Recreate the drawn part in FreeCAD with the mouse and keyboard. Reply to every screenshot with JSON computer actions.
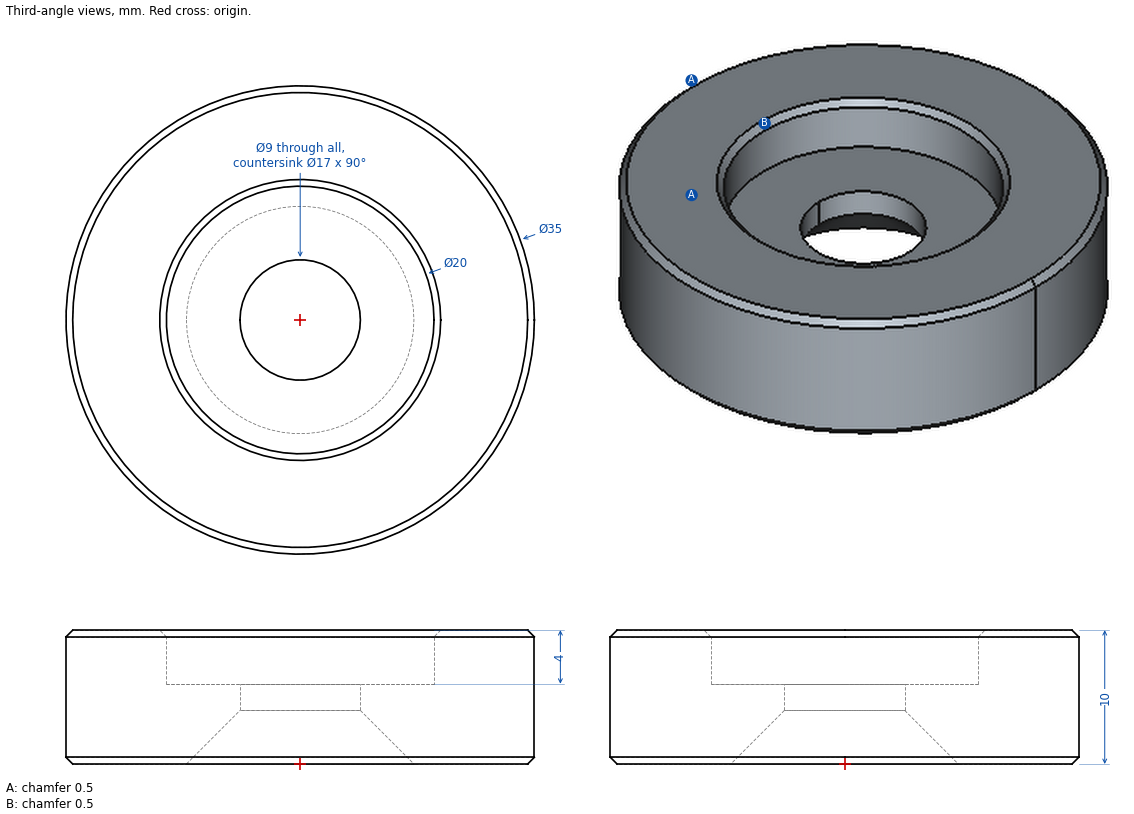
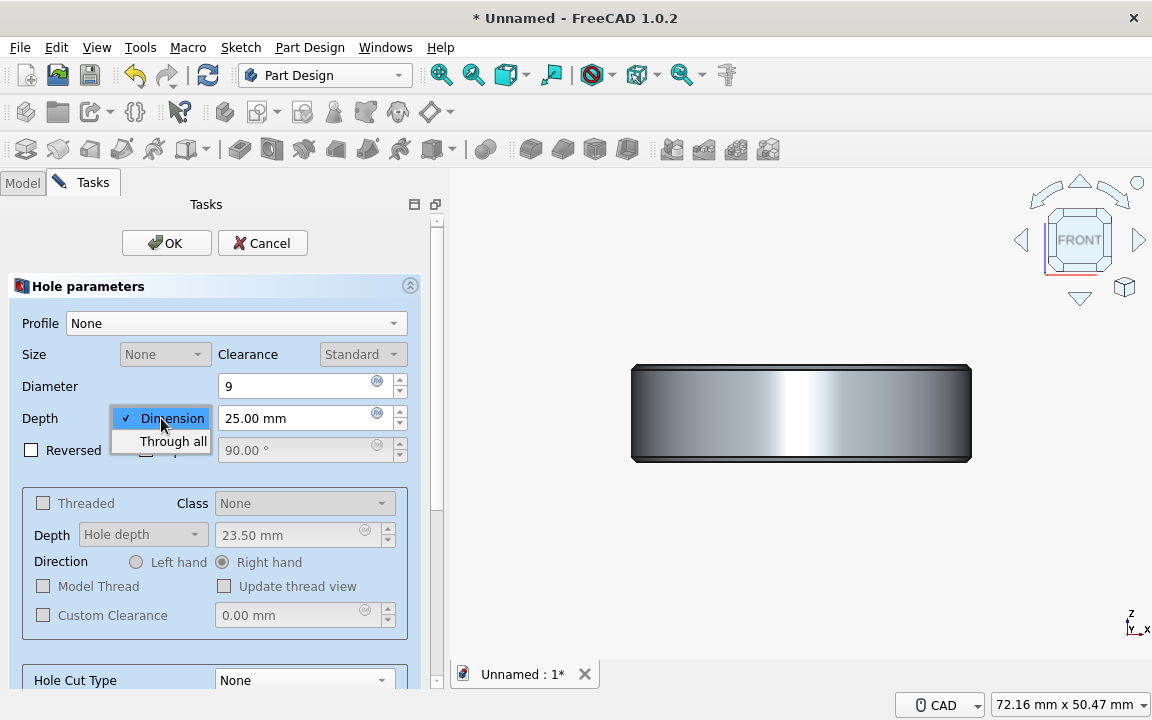
{"action": "left_click", "coordinate": [160, 442]}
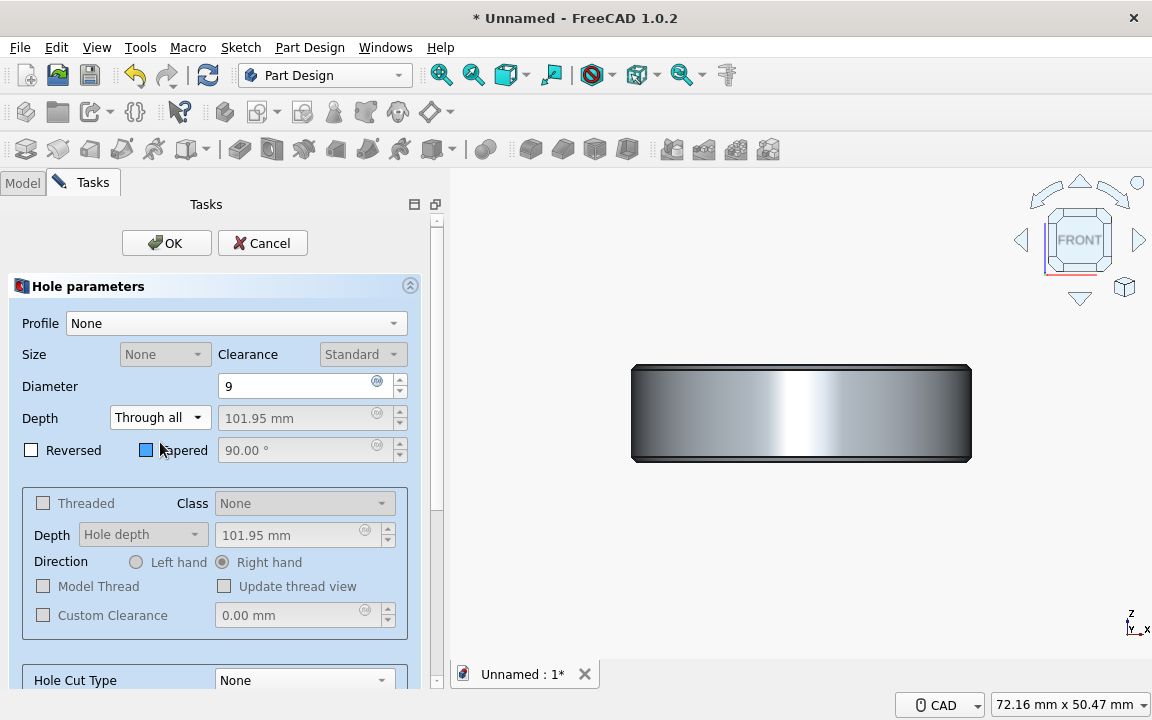
{"action": "left_click", "coordinate": [30, 450]}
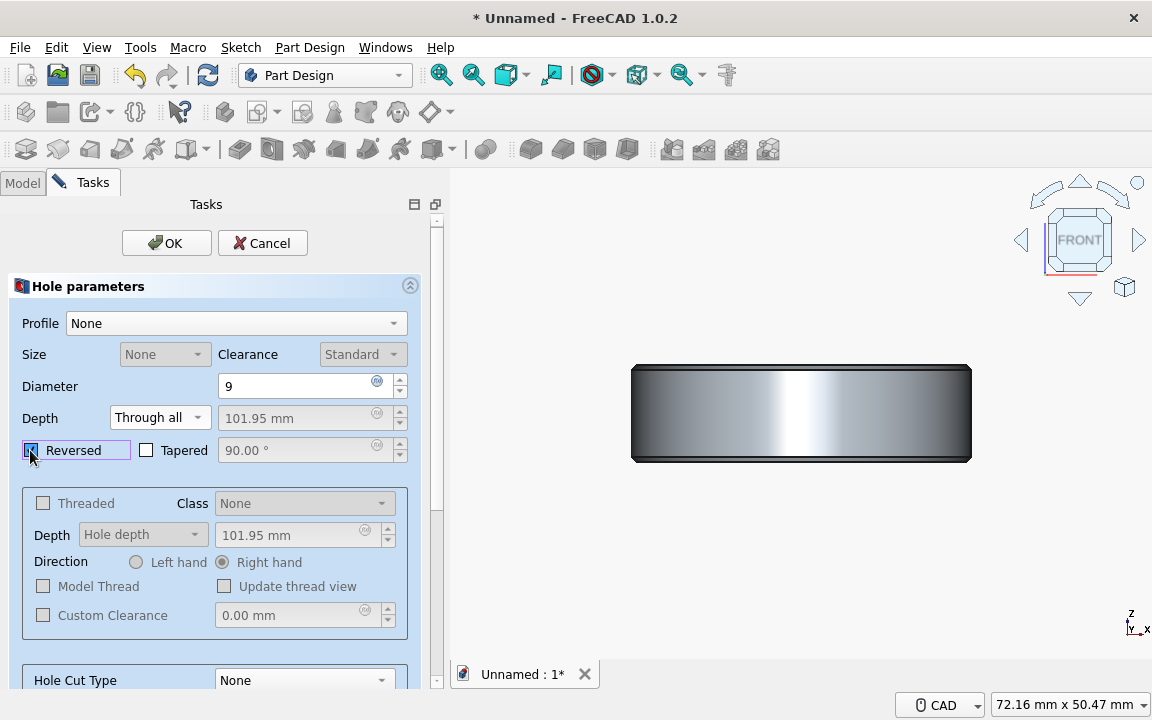
{"action": "scroll", "coordinate": [437, 451], "scroll_direction": "down", "scroll_amount": 2}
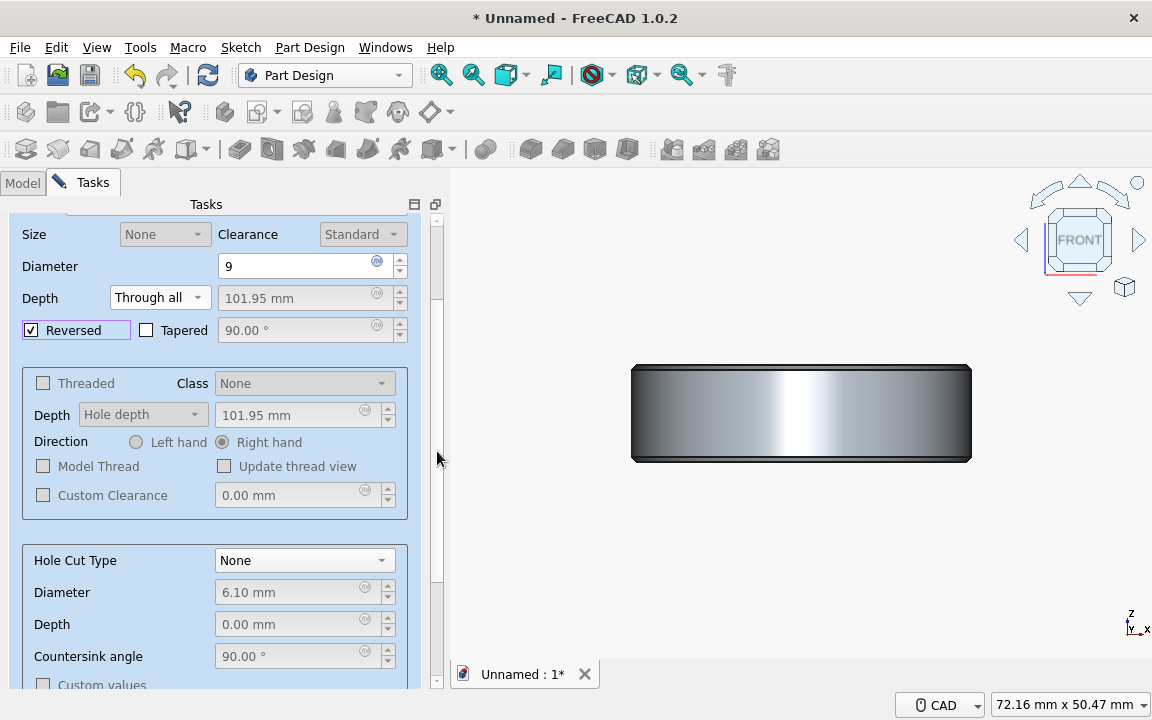
{"action": "left_click", "coordinate": [306, 560]}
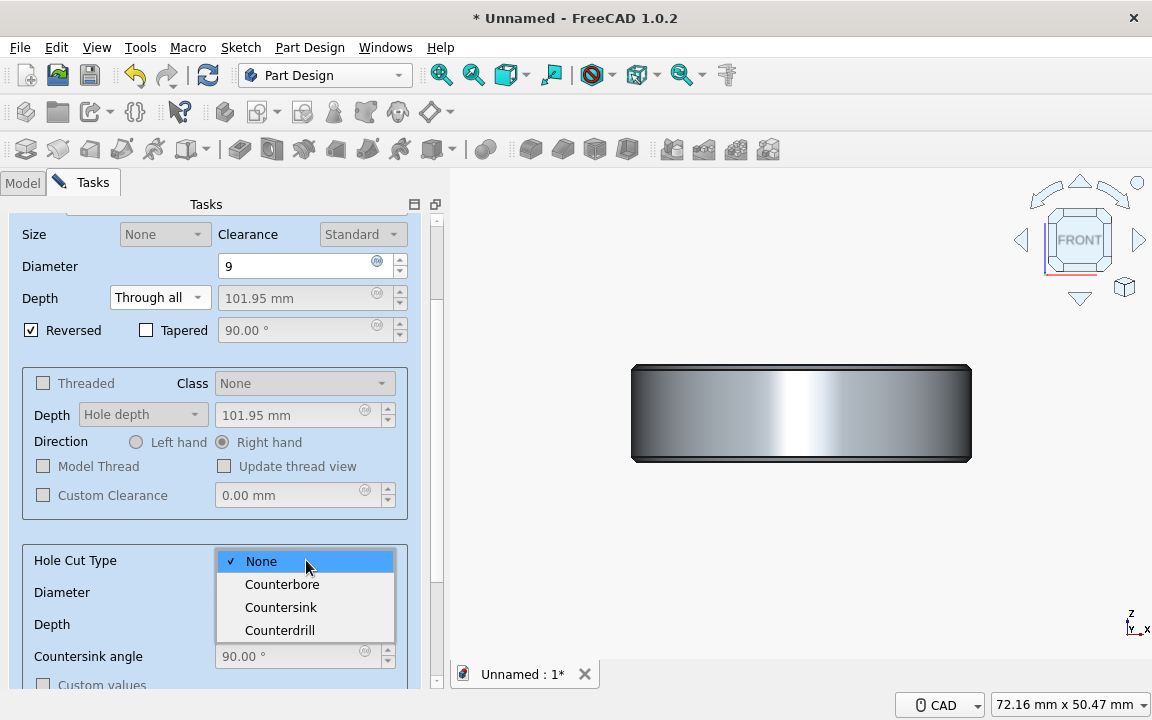
{"action": "left_click", "coordinate": [304, 608]}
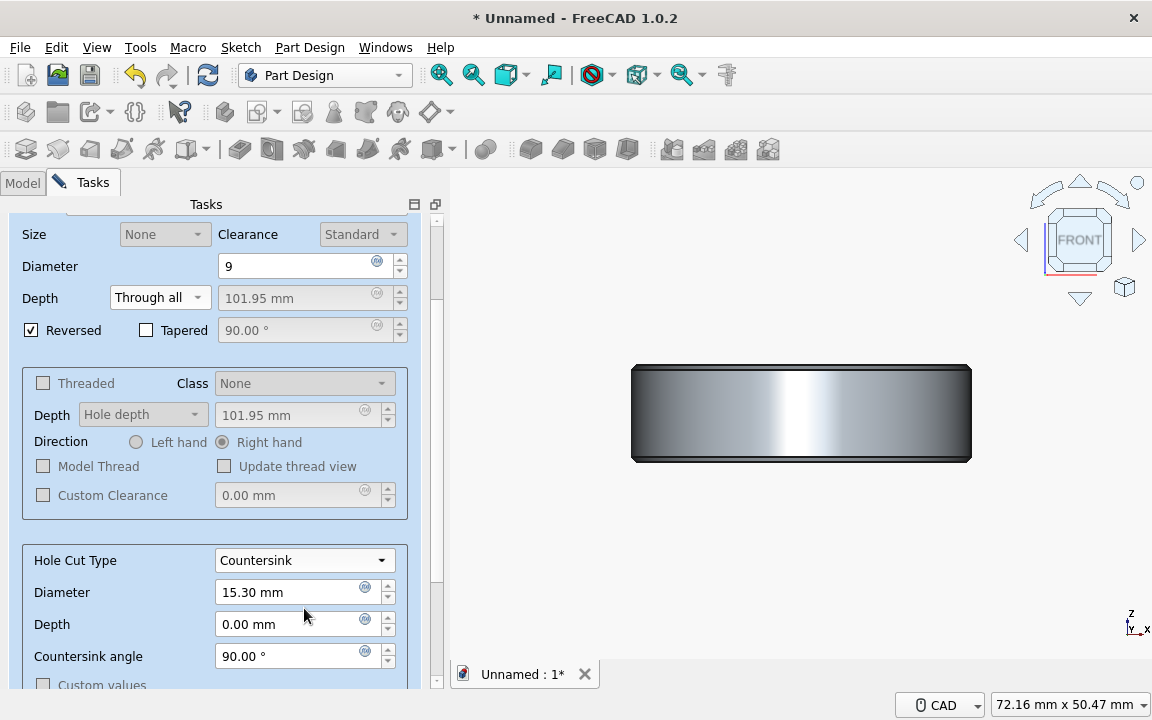
{"action": "triple_click", "coordinate": [298, 592]}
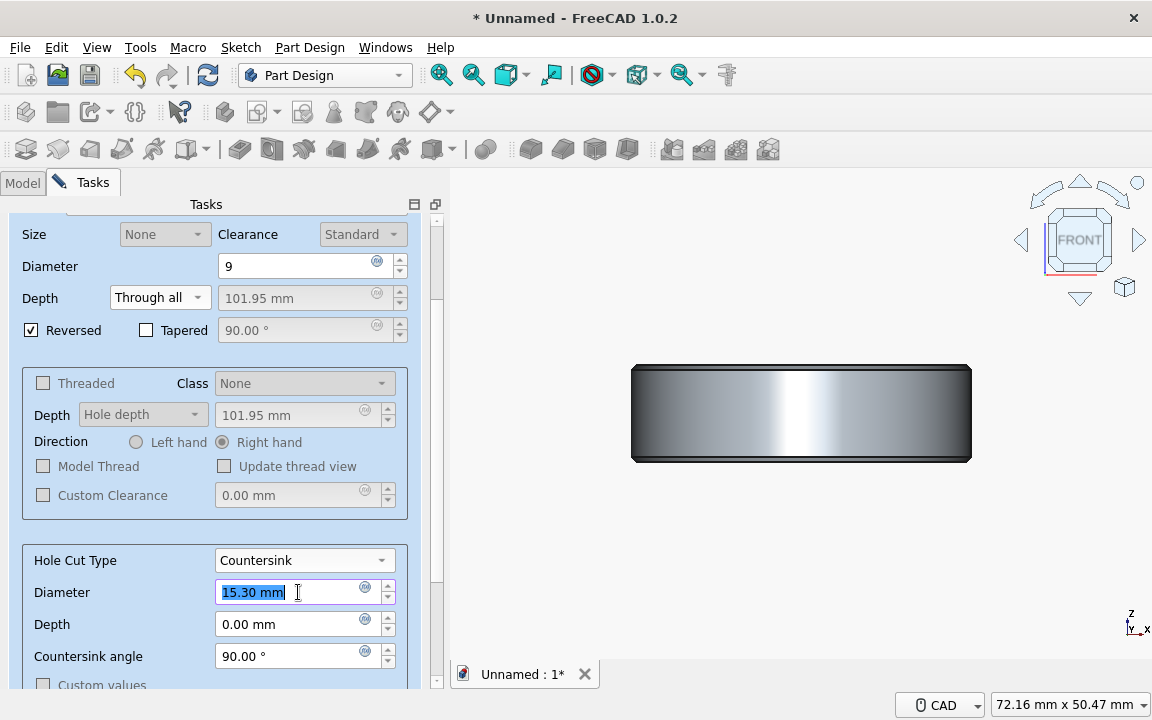
{"action": "type", "text": "17"}
{"action": "key", "text": "Tab"}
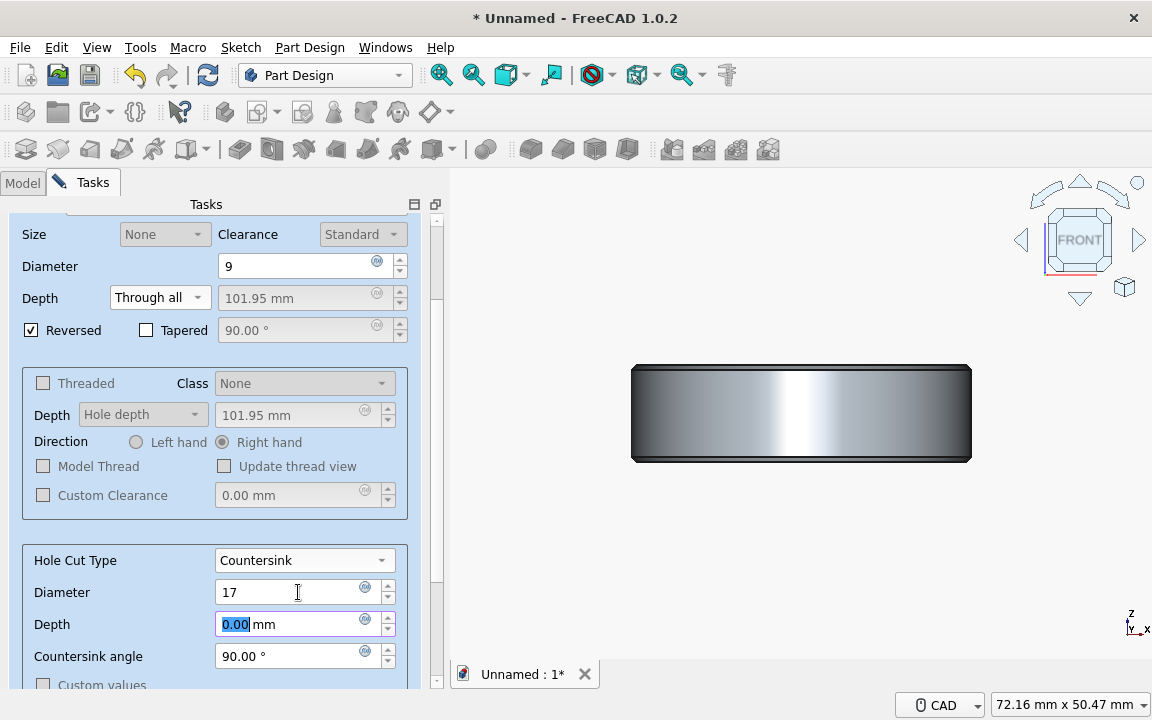
{"action": "scroll", "coordinate": [437, 451], "scroll_direction": "up", "scroll_amount": 3}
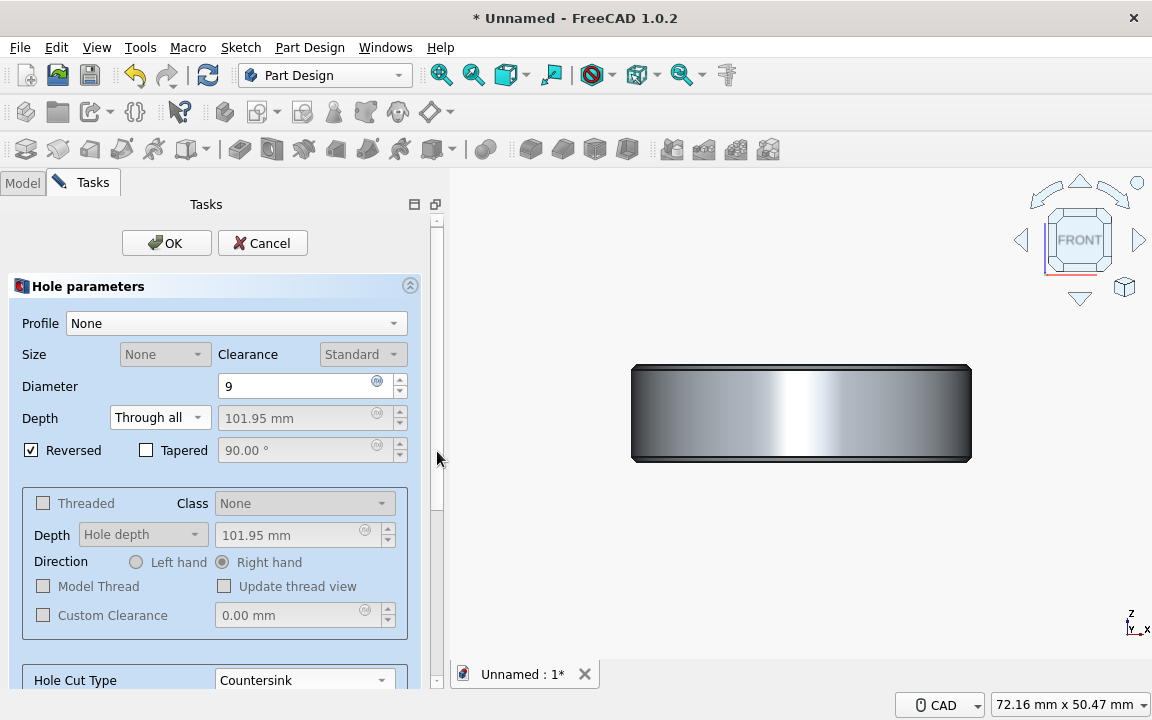
{"action": "left_click", "coordinate": [167, 243]}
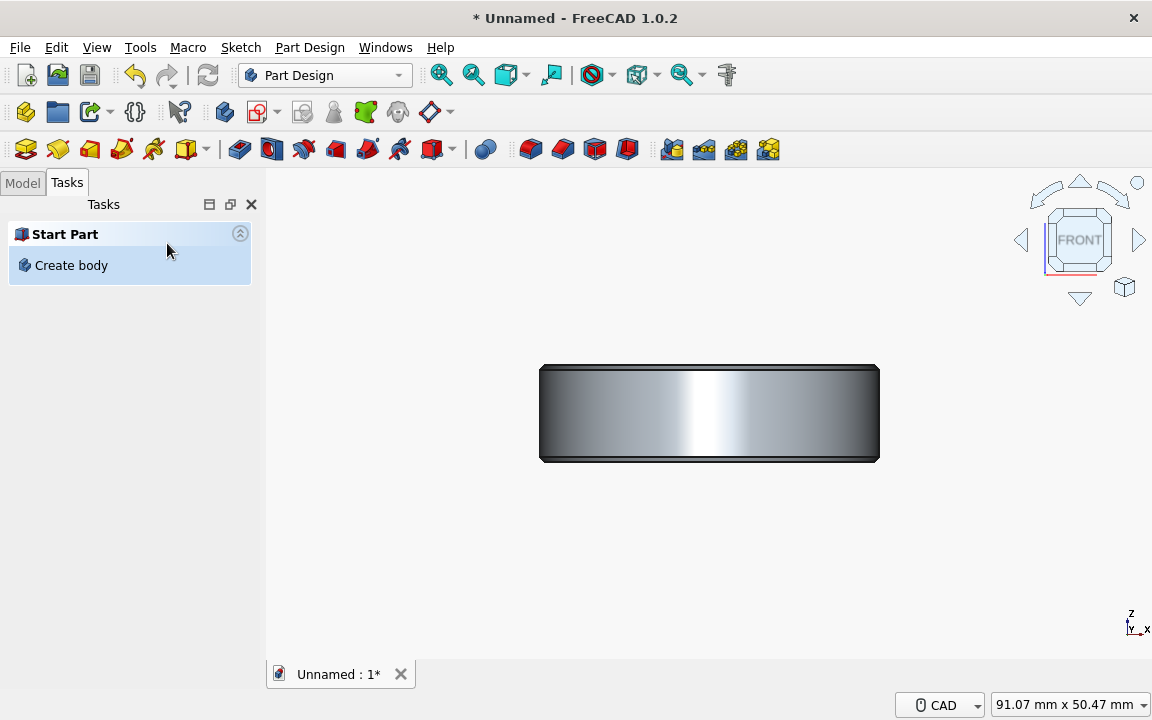
{"action": "left_click", "coordinate": [442, 76]}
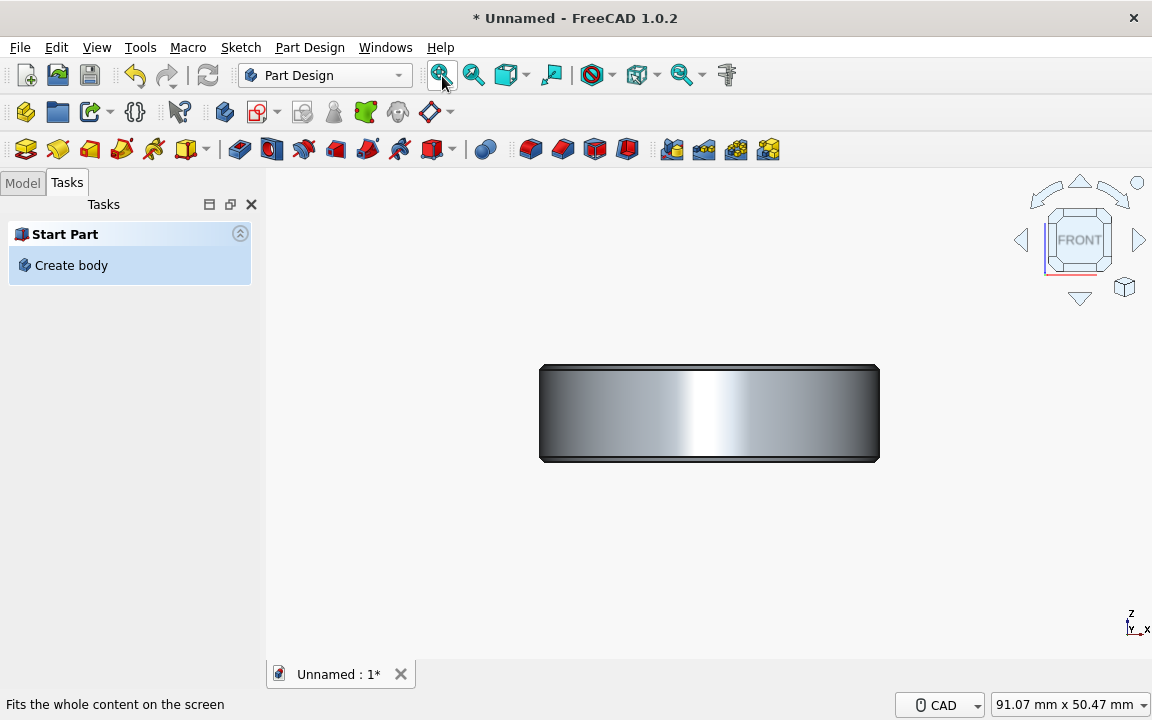
{"action": "key", "text": "0"}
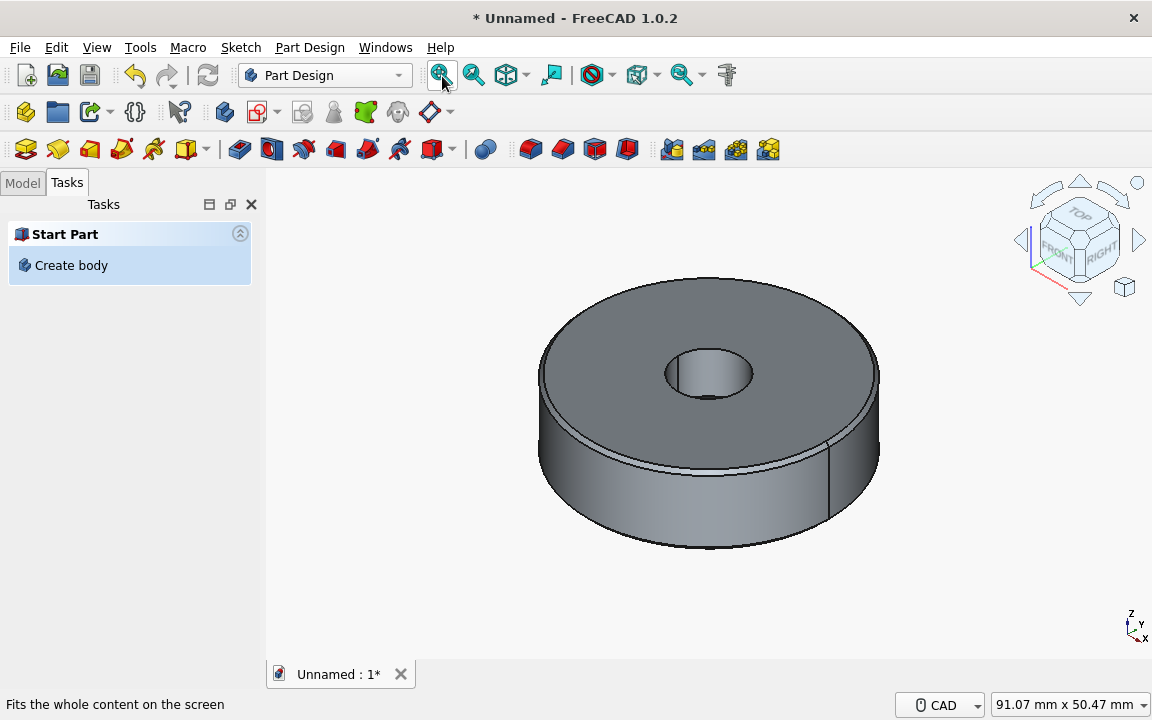
{"action": "left_click", "coordinate": [675, 431]}